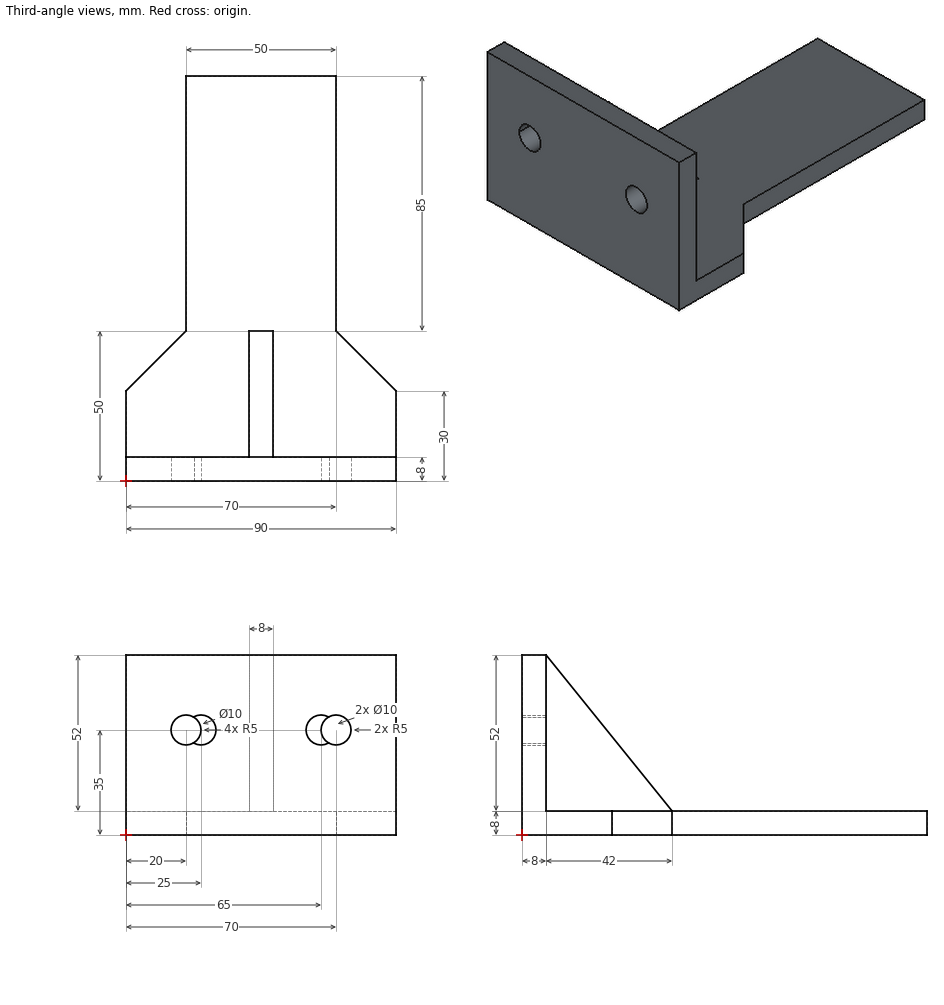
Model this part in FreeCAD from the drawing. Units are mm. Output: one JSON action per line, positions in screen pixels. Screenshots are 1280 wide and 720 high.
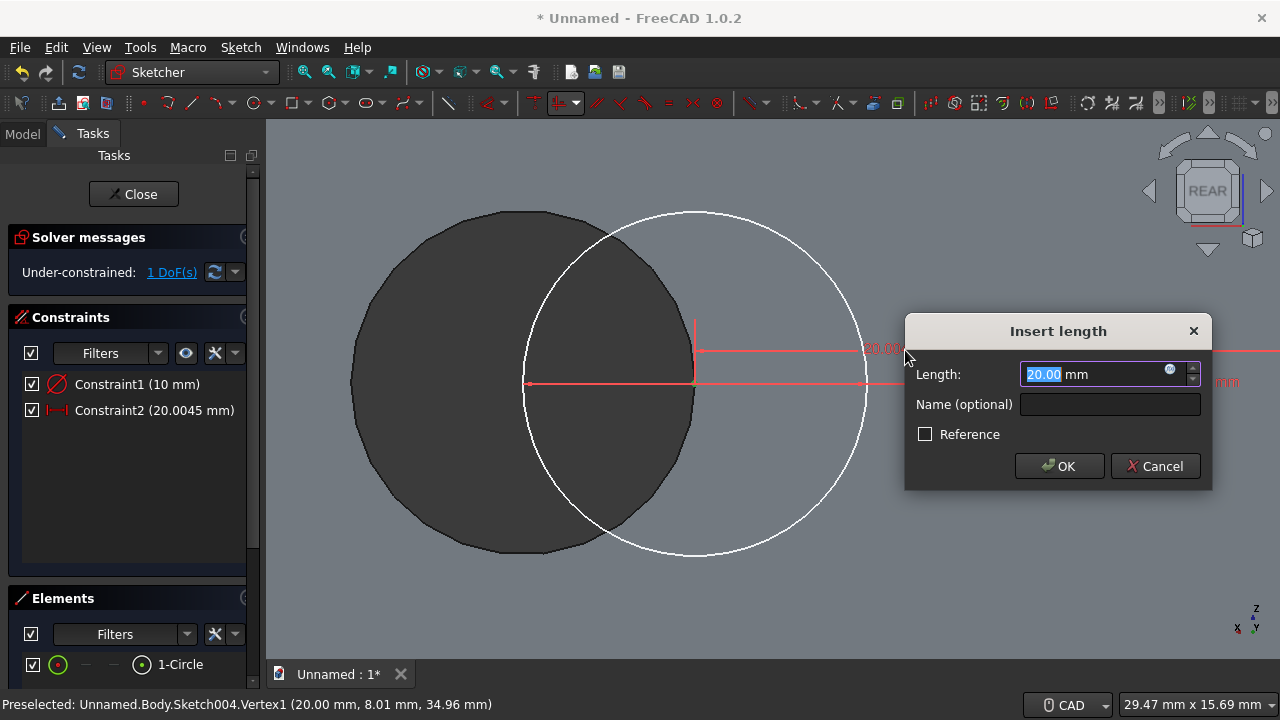
{"action": "type", "text": "20"}
{"action": "key", "text": "Return"}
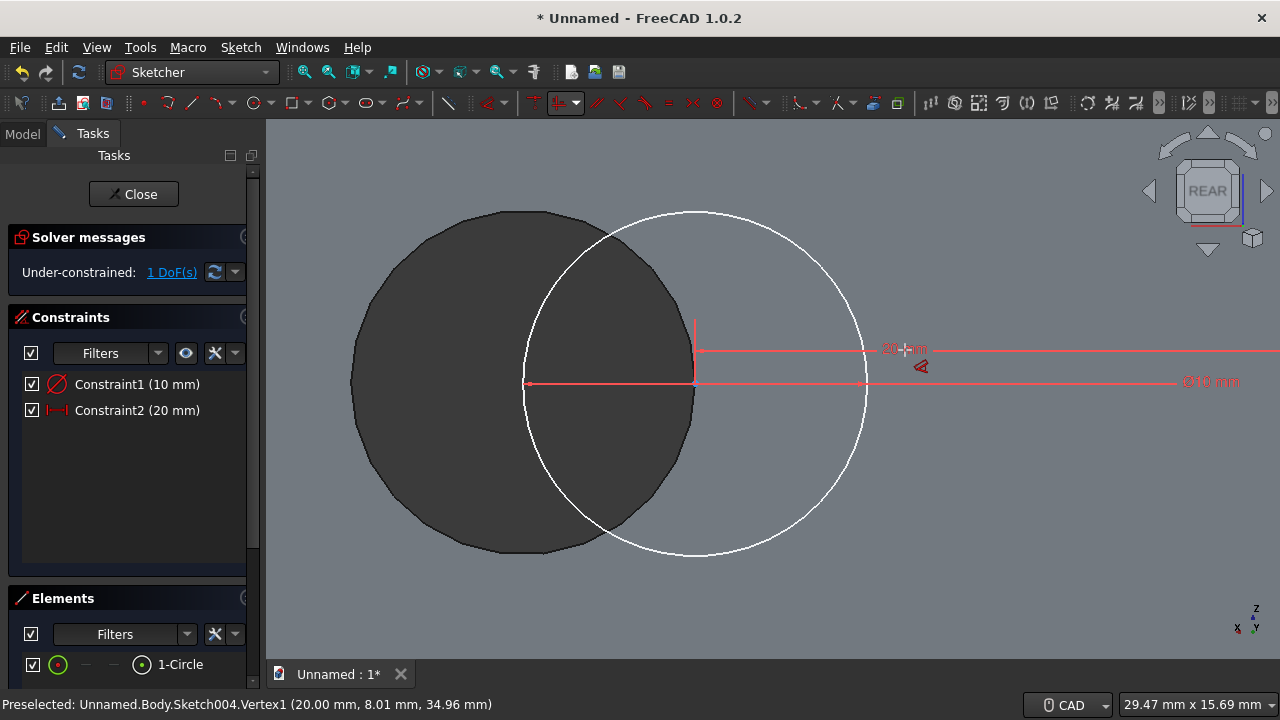
{"action": "left_click", "coordinate": [695, 384]}
{"action": "left_click", "coordinate": [661, 508]}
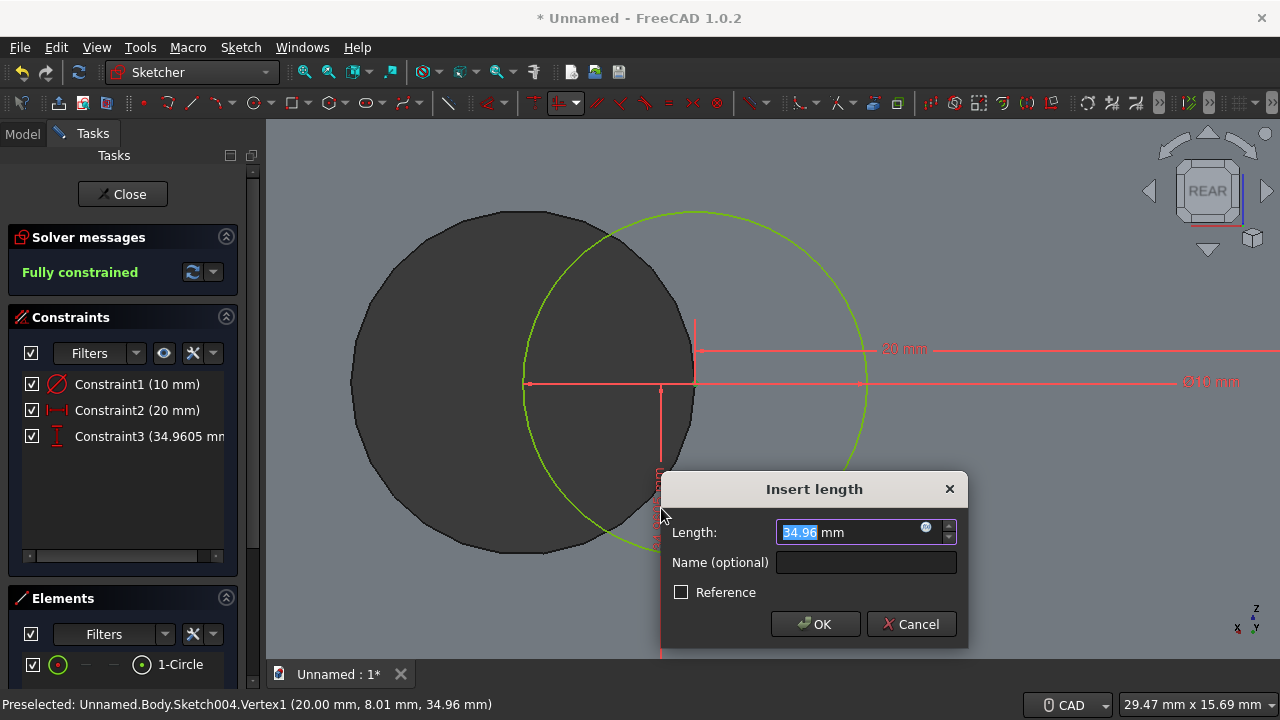
{"action": "type", "text": "35"}
{"action": "key", "text": "Return"}
{"action": "key", "text": "Escape"}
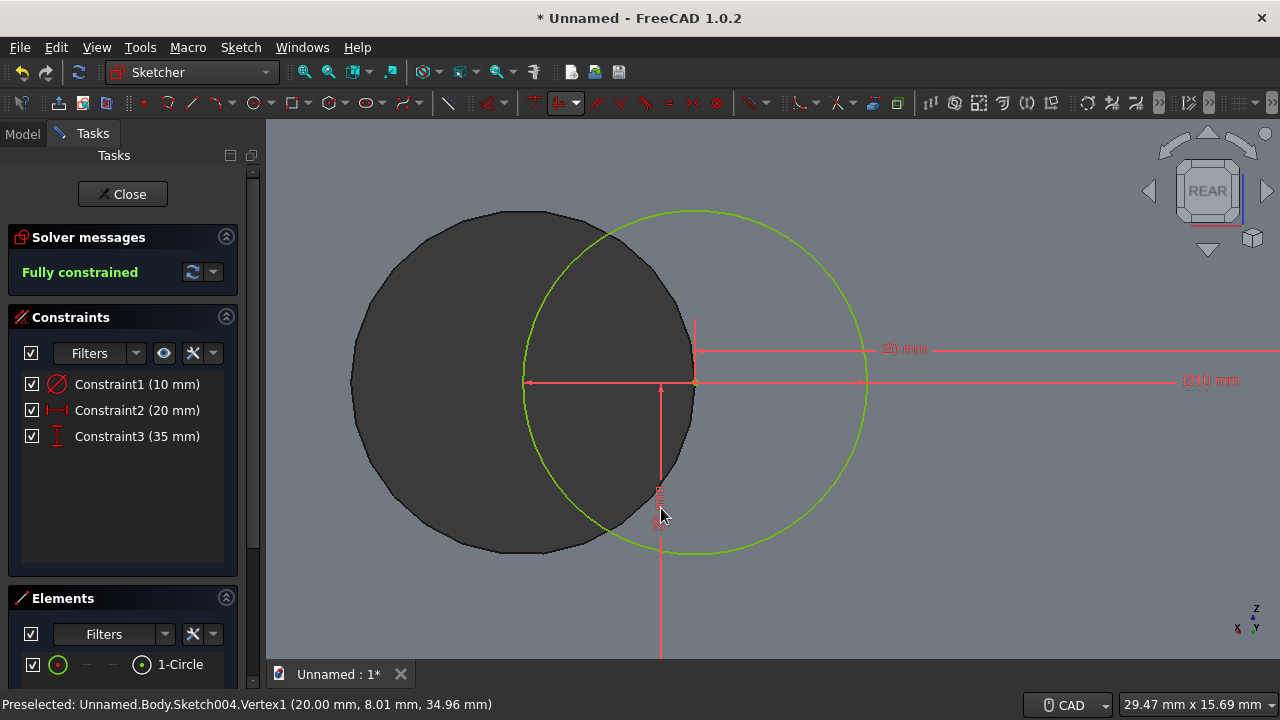
{"action": "left_click", "coordinate": [123, 194]}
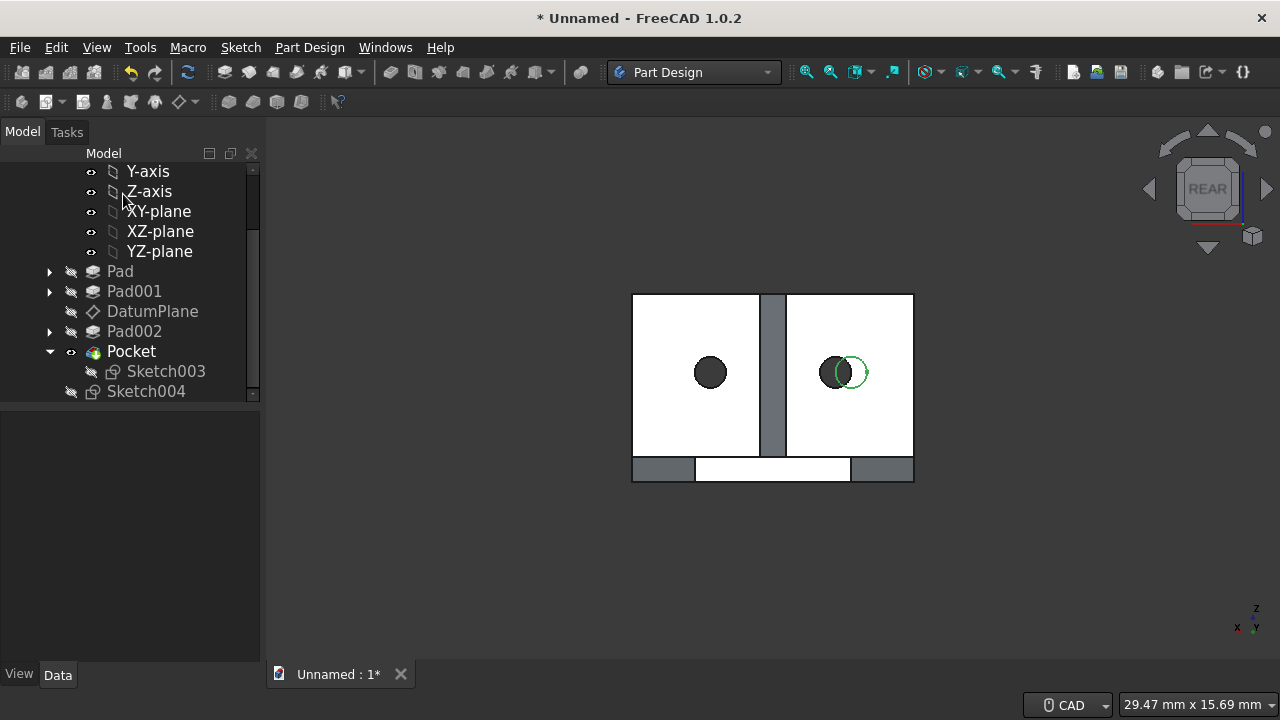
{"action": "left_click", "coordinate": [392, 72]}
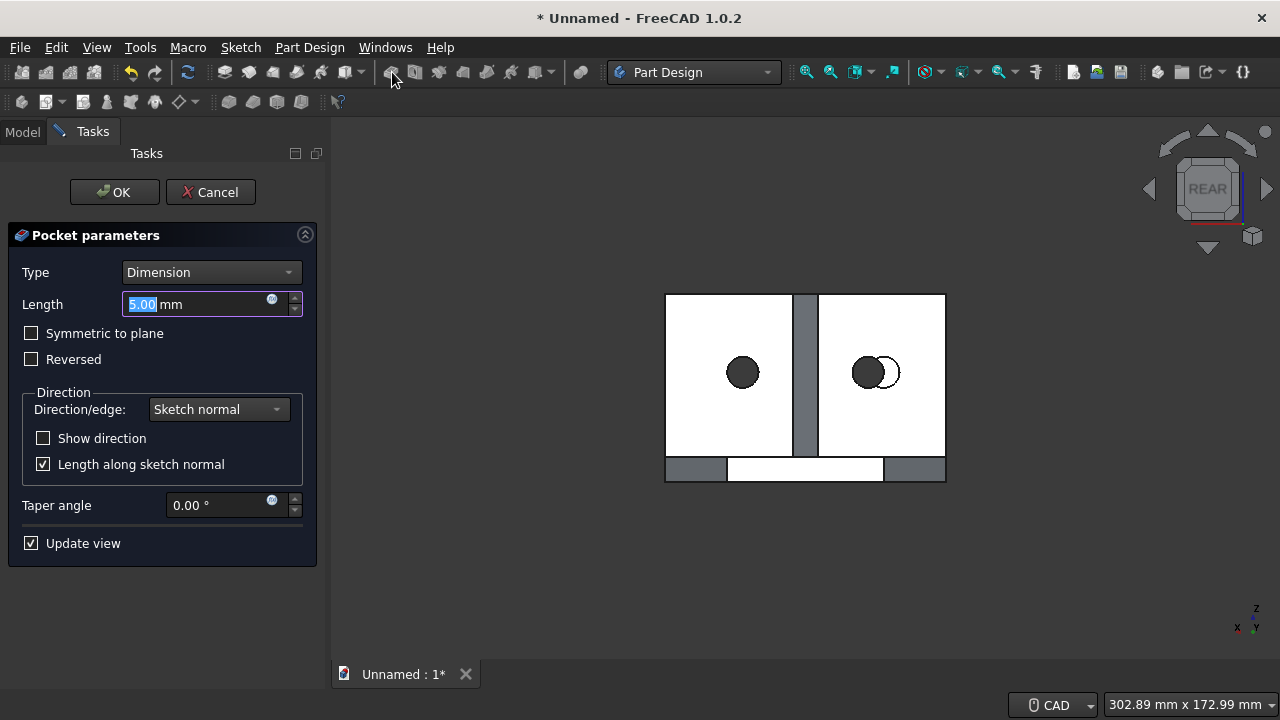
{"action": "type", "text": "10"}
{"action": "key", "text": "Tab"}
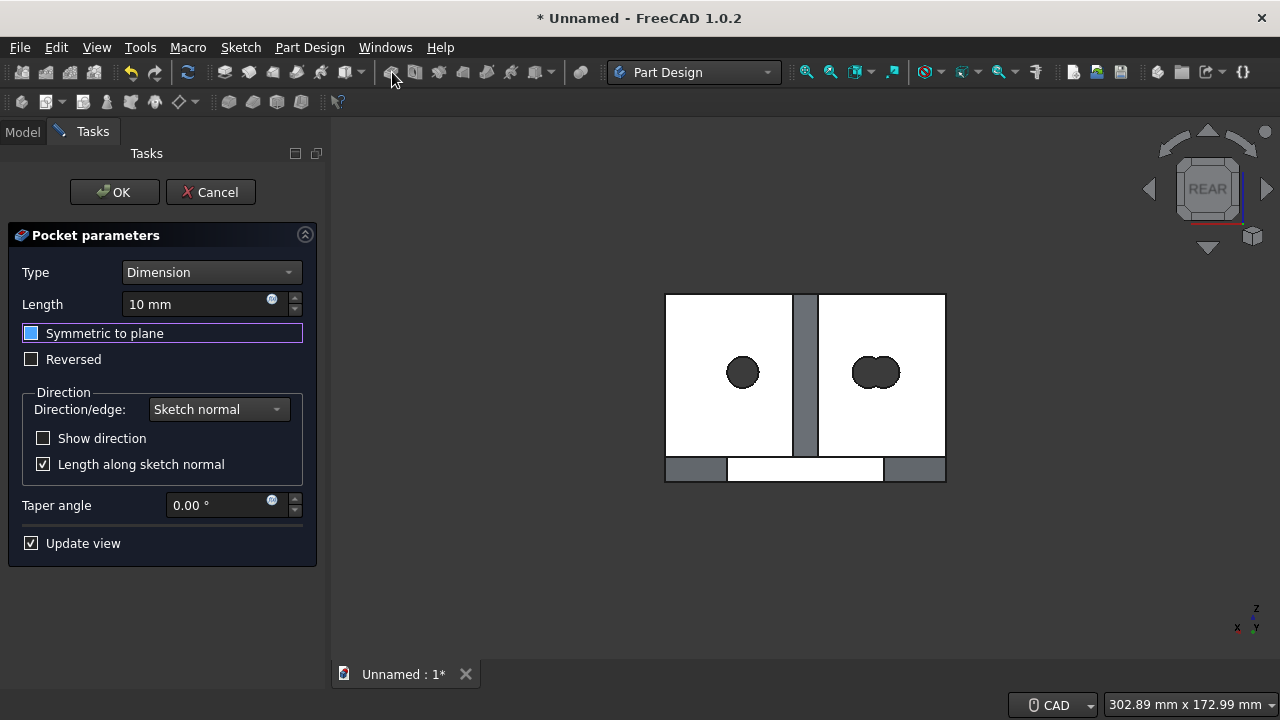
{"action": "left_click", "coordinate": [115, 192]}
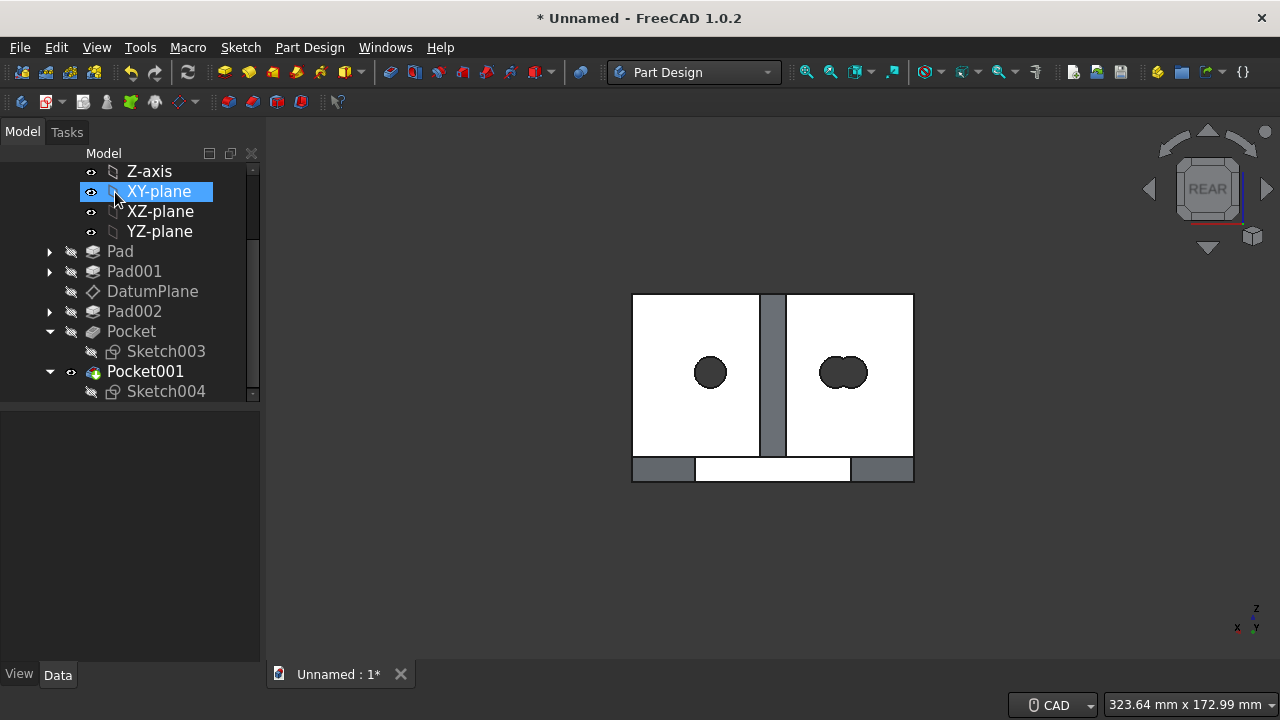
{"action": "left_click", "coordinate": [808, 72]}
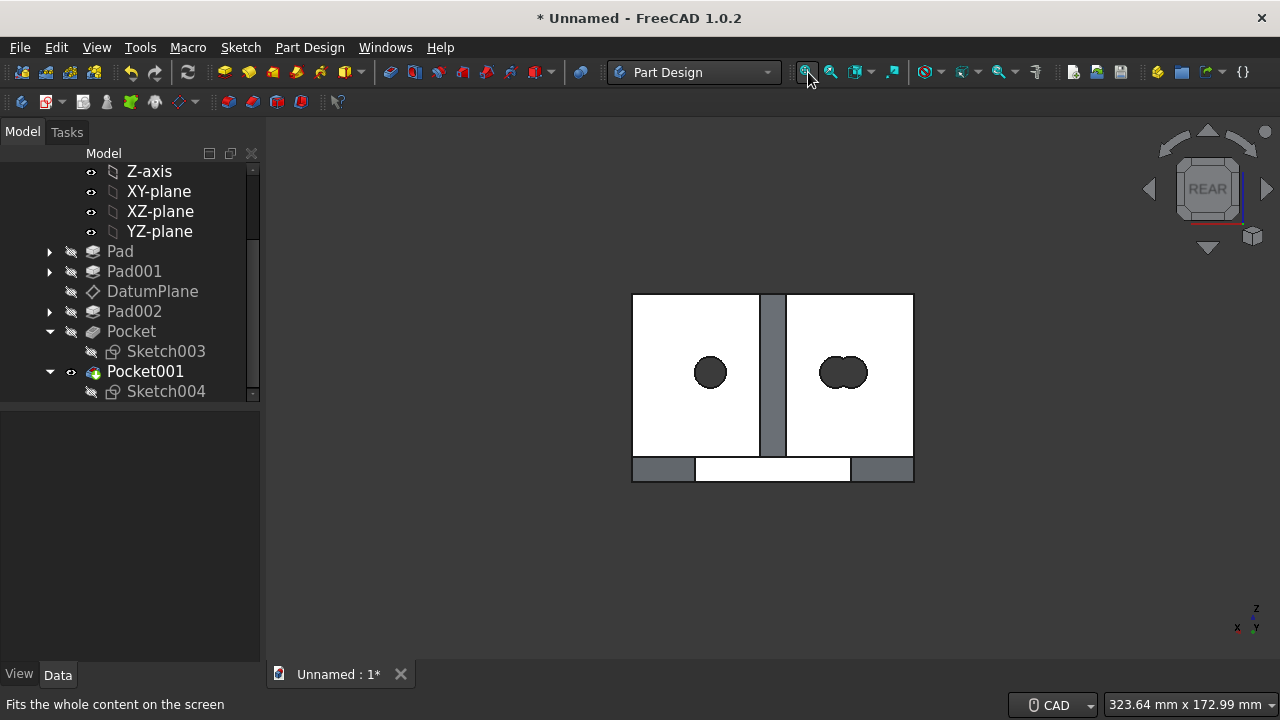
{"action": "left_click", "coordinate": [678, 421]}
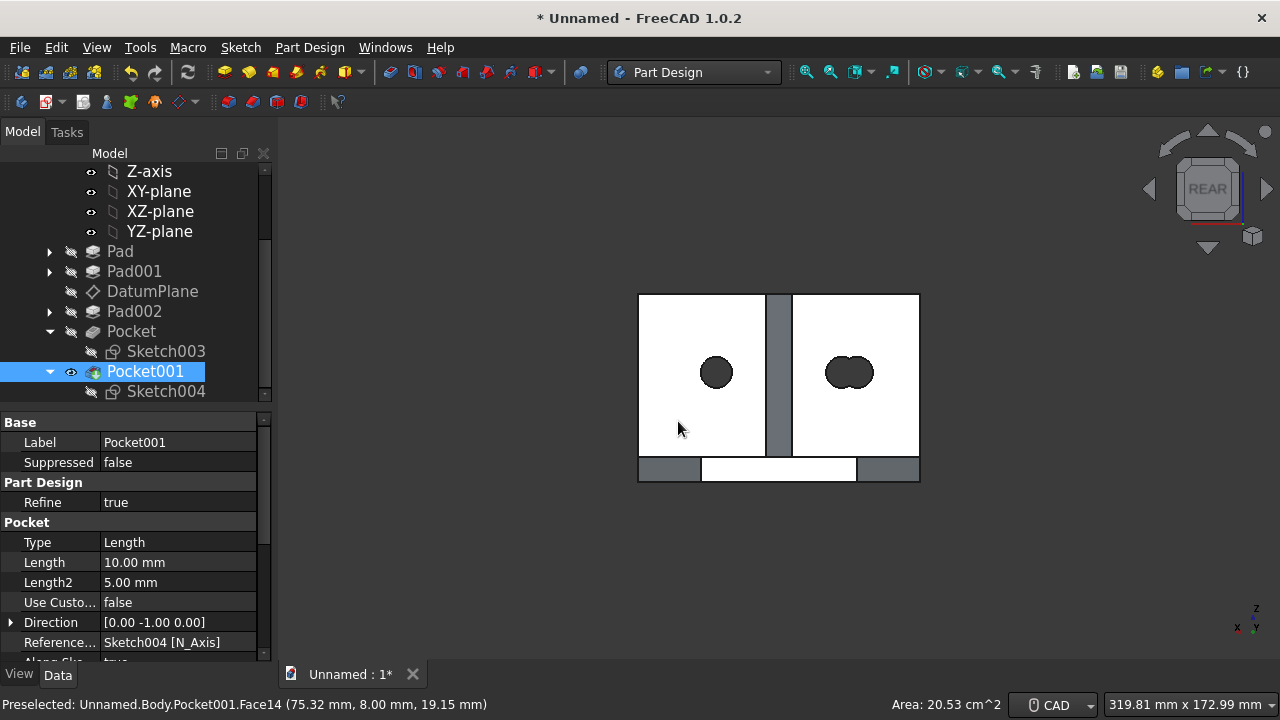
{"action": "left_click", "coordinate": [46, 102]}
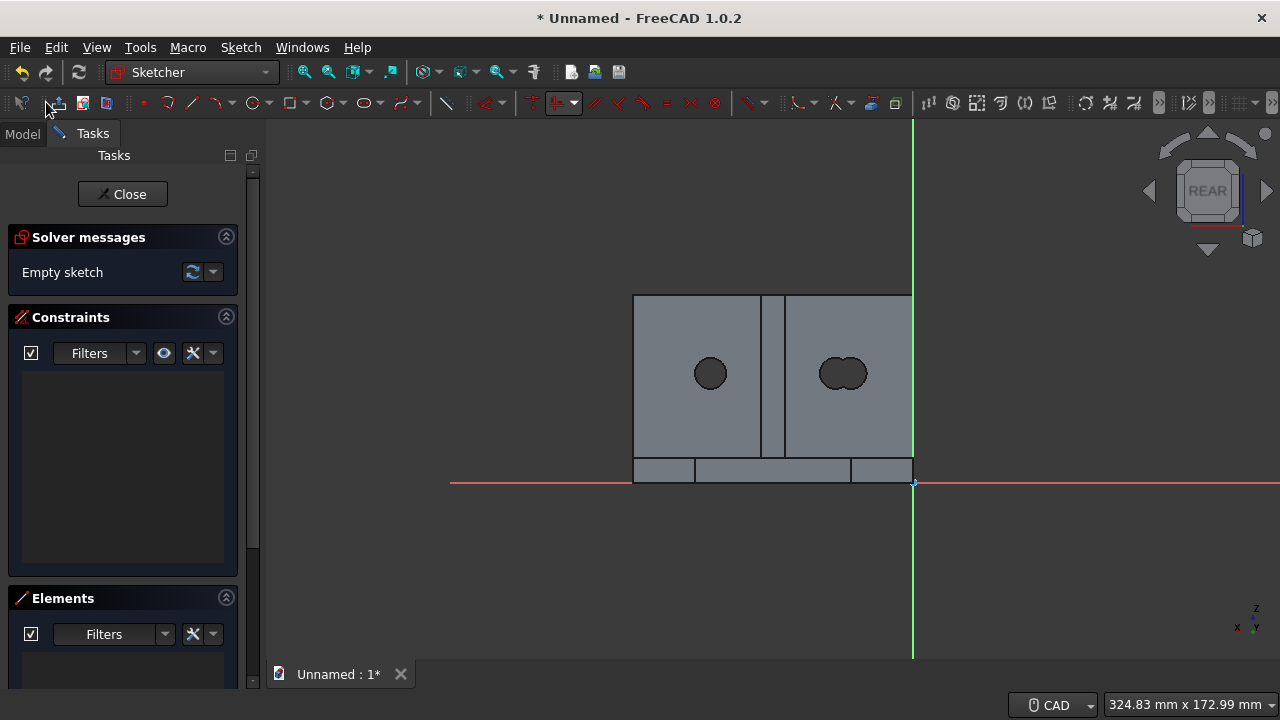
{"action": "scroll", "coordinate": [703, 372], "scroll_direction": "up", "scroll_amount": 13}